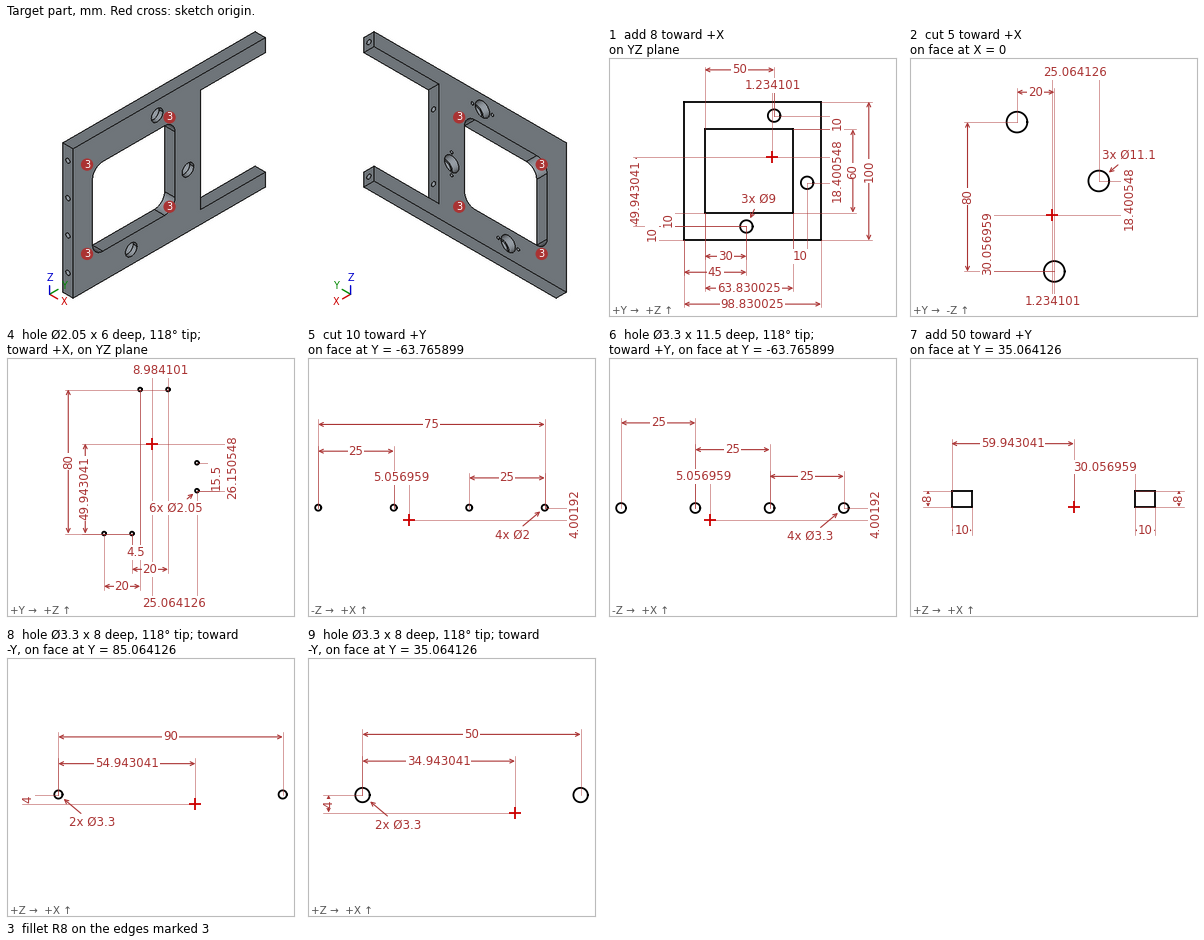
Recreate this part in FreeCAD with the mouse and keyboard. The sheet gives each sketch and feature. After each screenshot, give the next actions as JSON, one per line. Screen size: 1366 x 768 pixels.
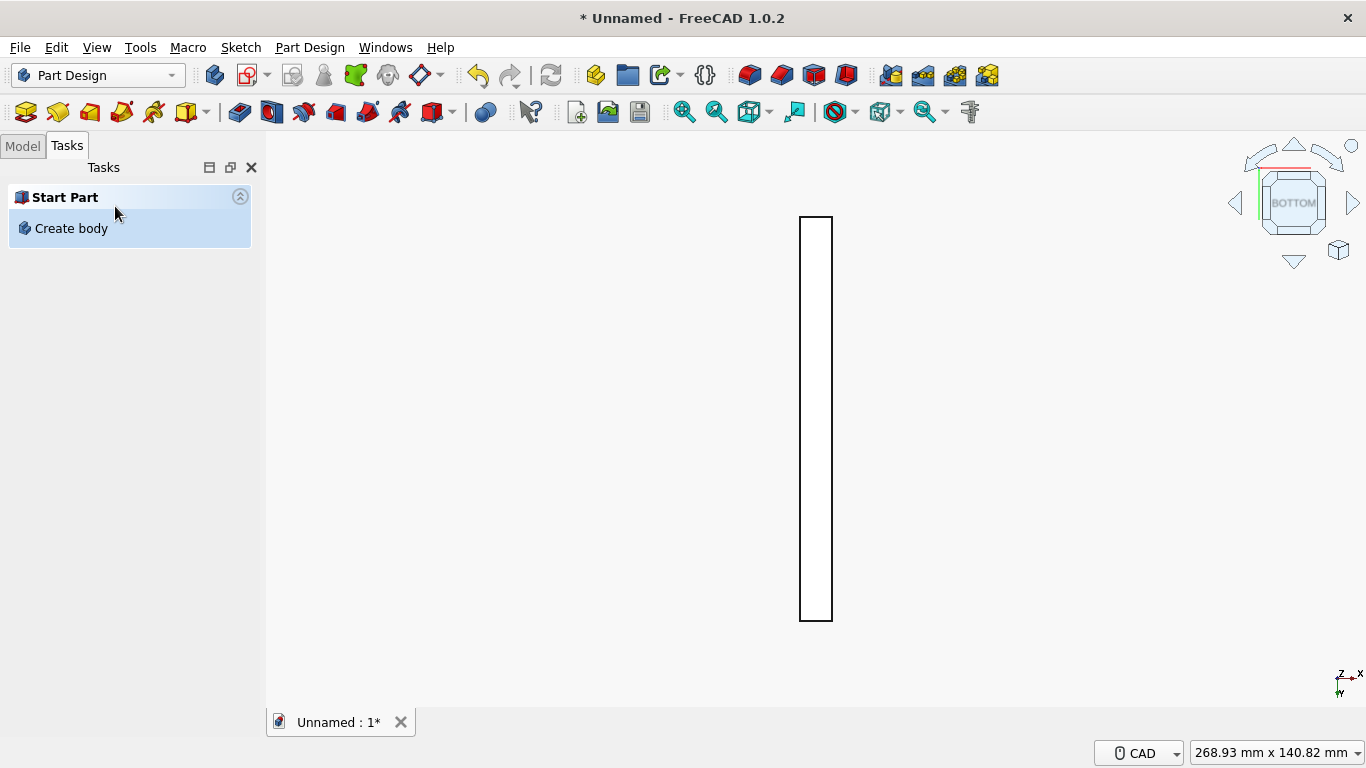
{"action": "key", "text": "4"}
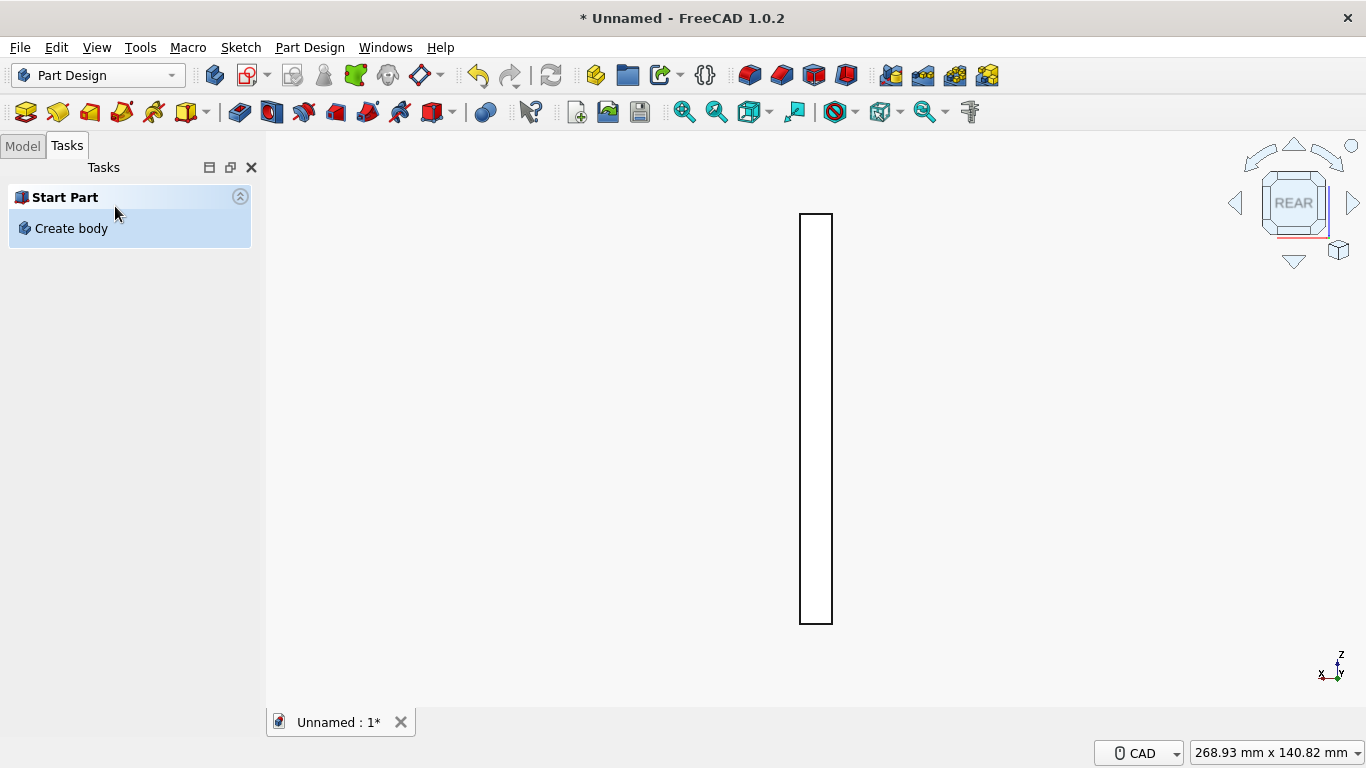
{"action": "key", "text": "6"}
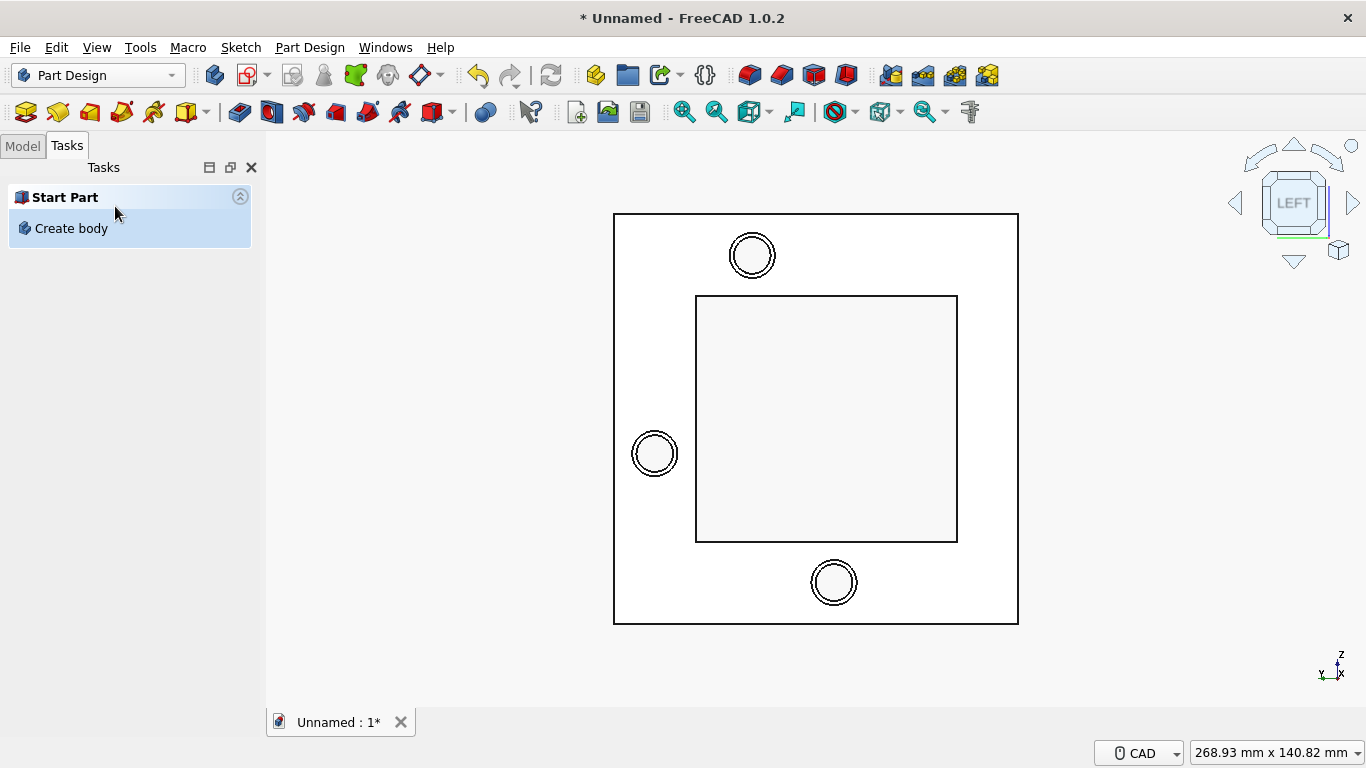
{"action": "key", "text": "v 3"}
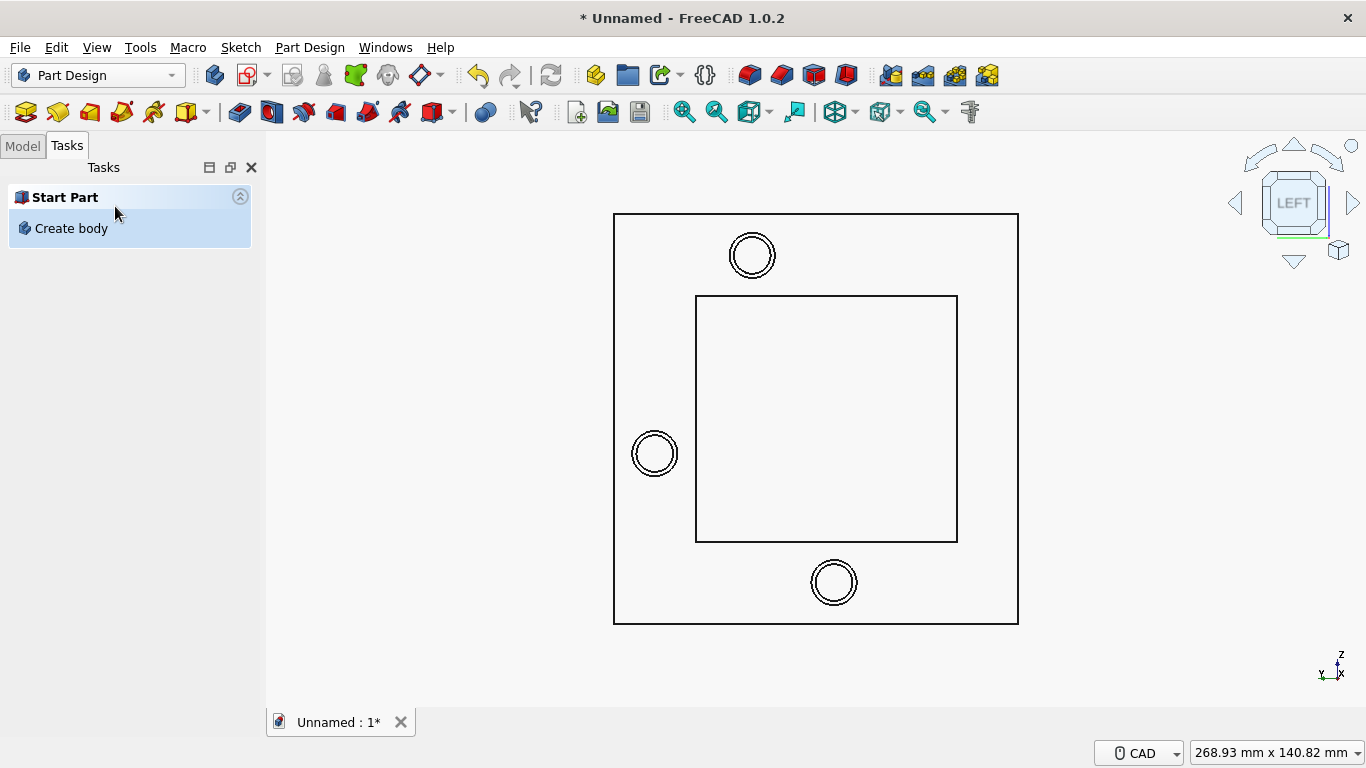
{"action": "key", "text": "0"}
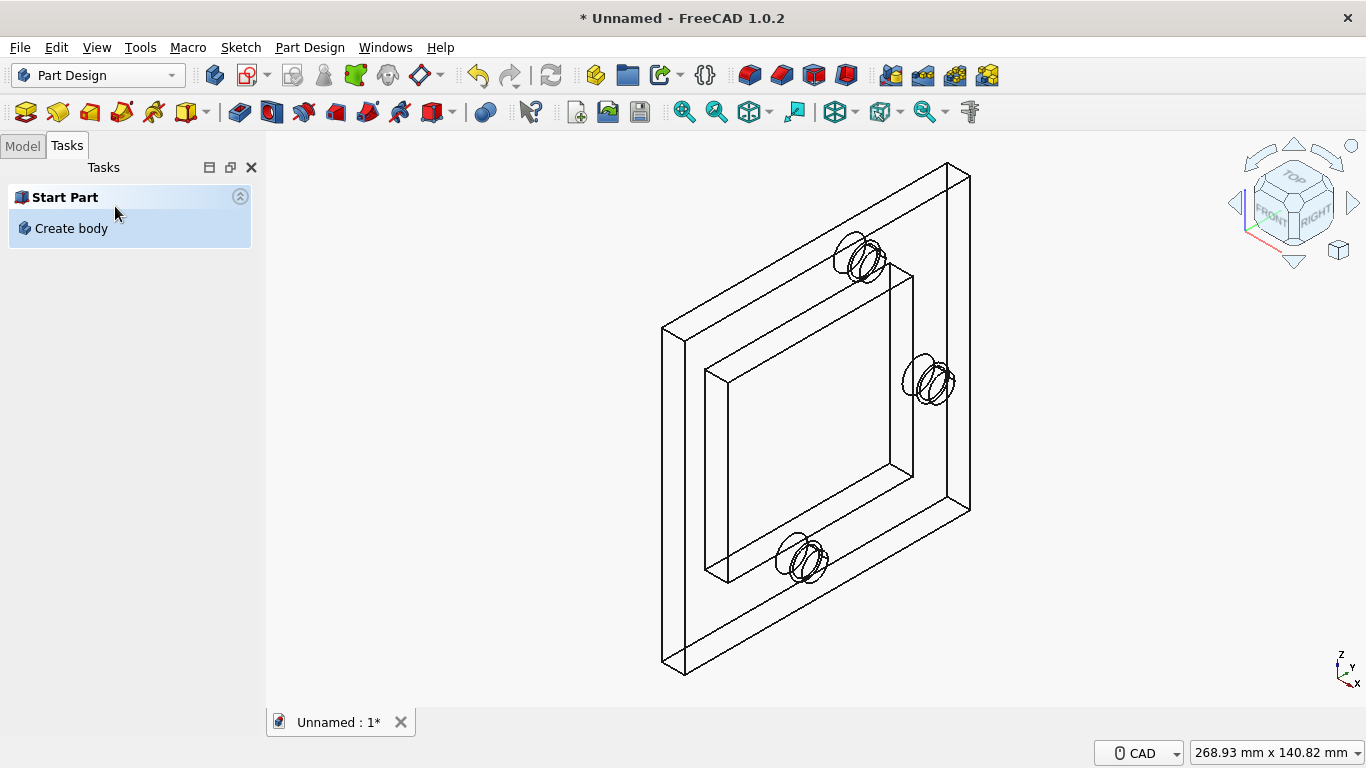
{"action": "left_click", "coordinate": [901, 269]}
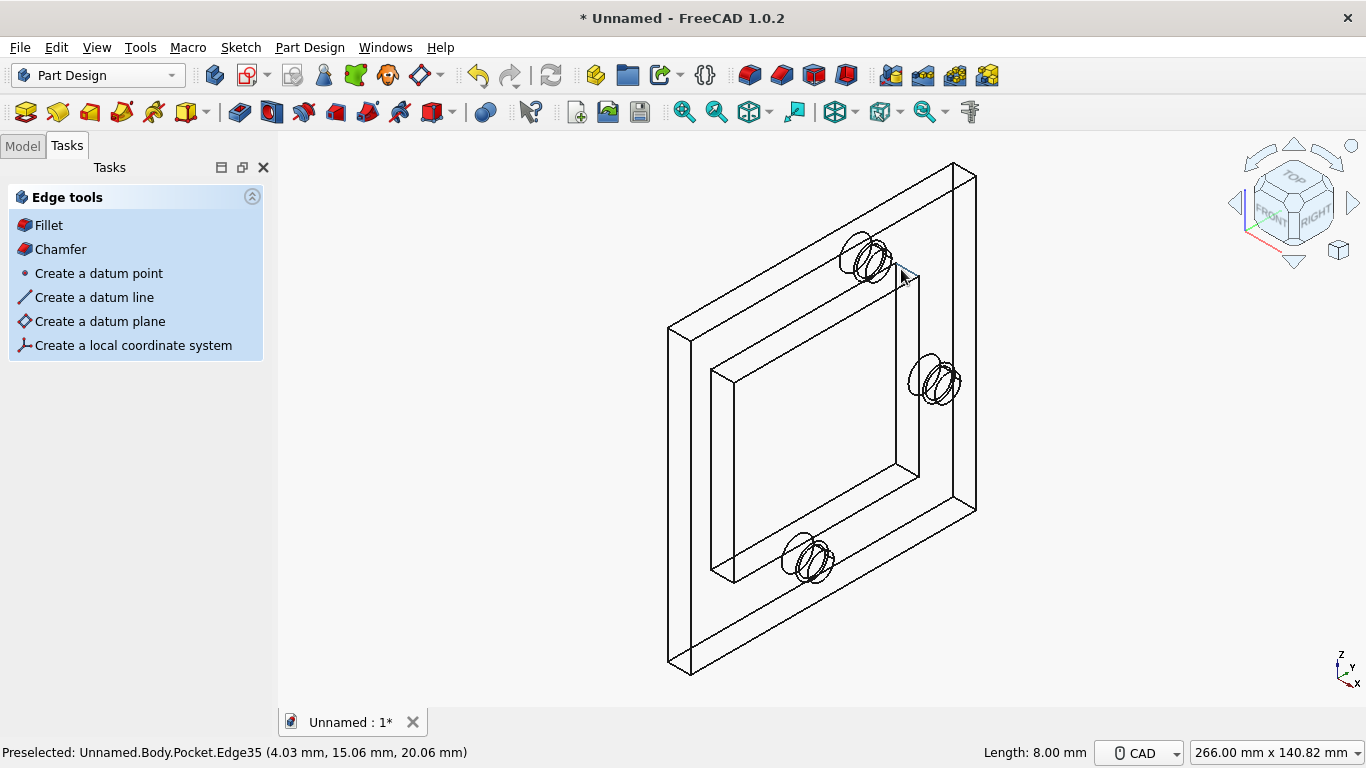
{"action": "left_click", "coordinate": [722, 375], "text": "ctrl"}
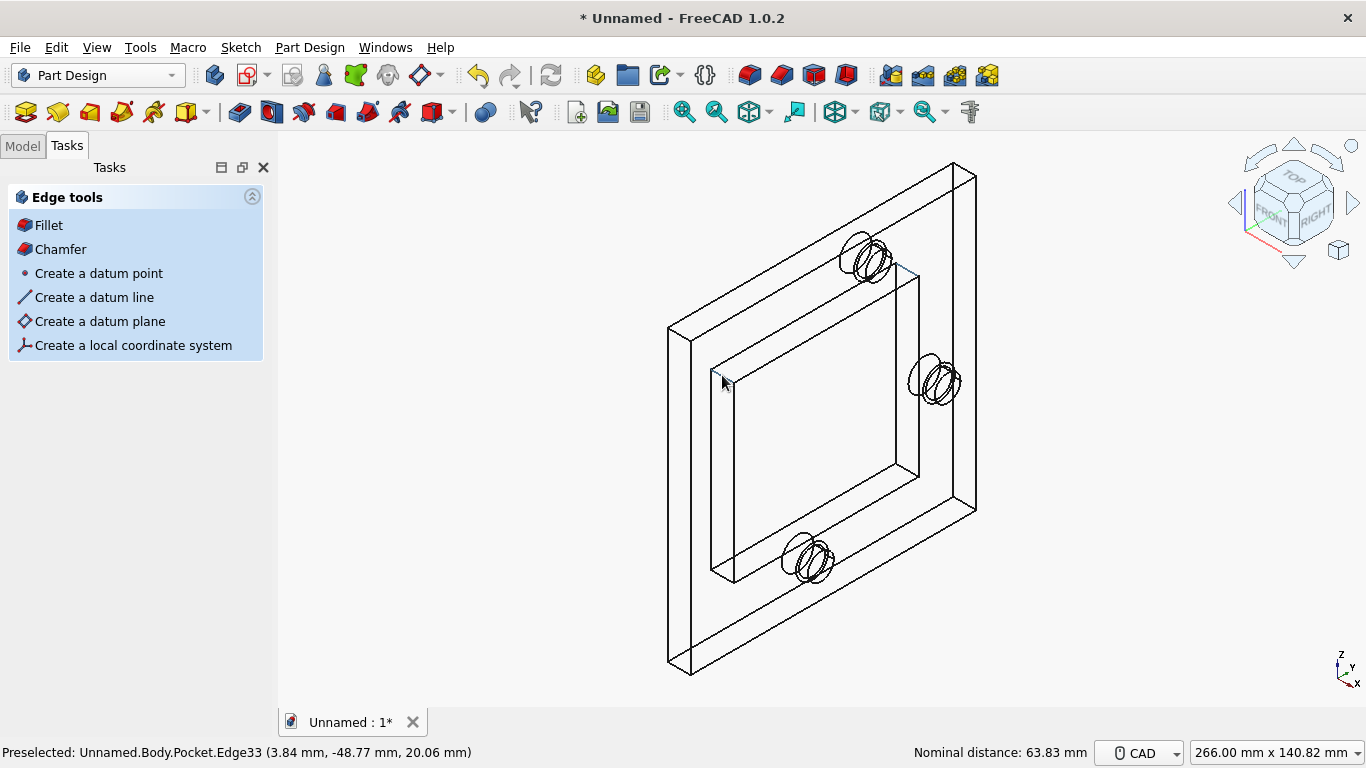
{"action": "left_click", "coordinate": [722, 576], "text": "ctrl"}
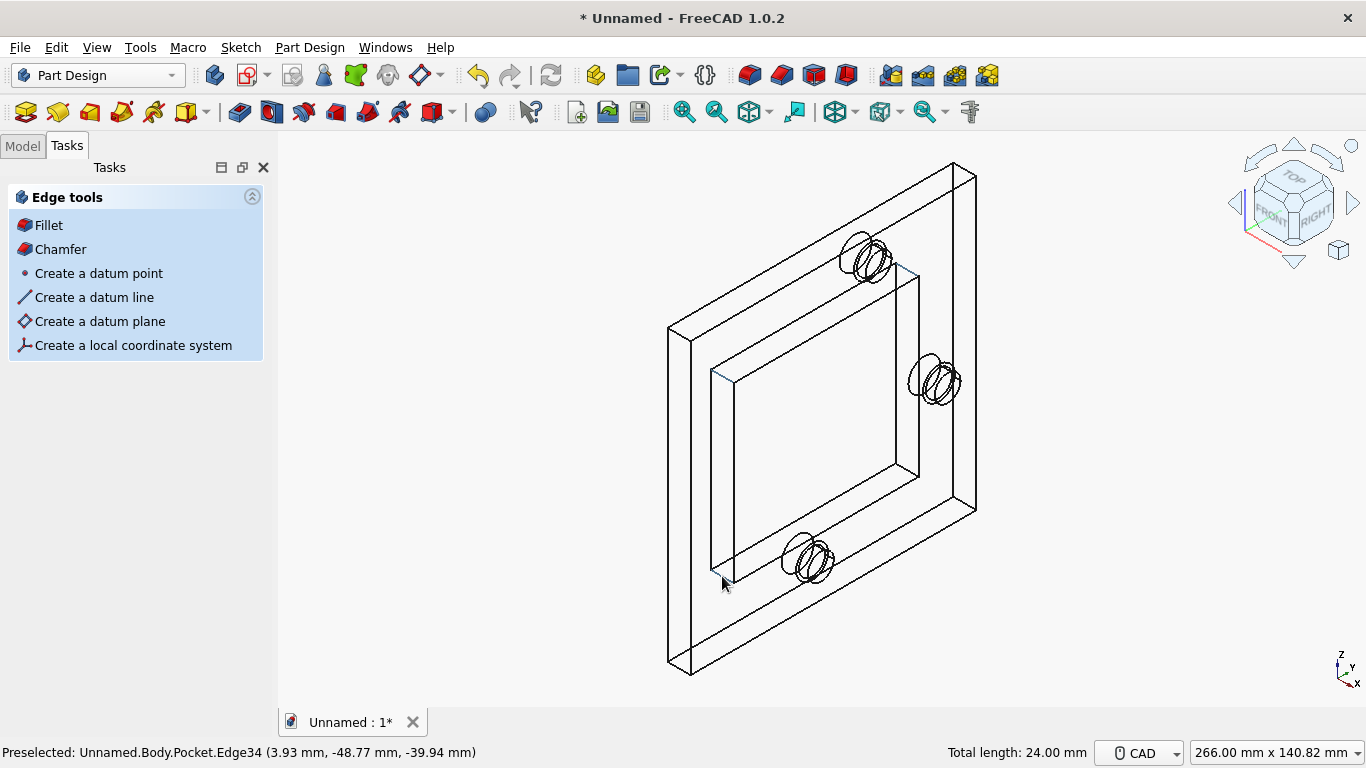
{"action": "left_click", "coordinate": [907, 469], "text": "ctrl"}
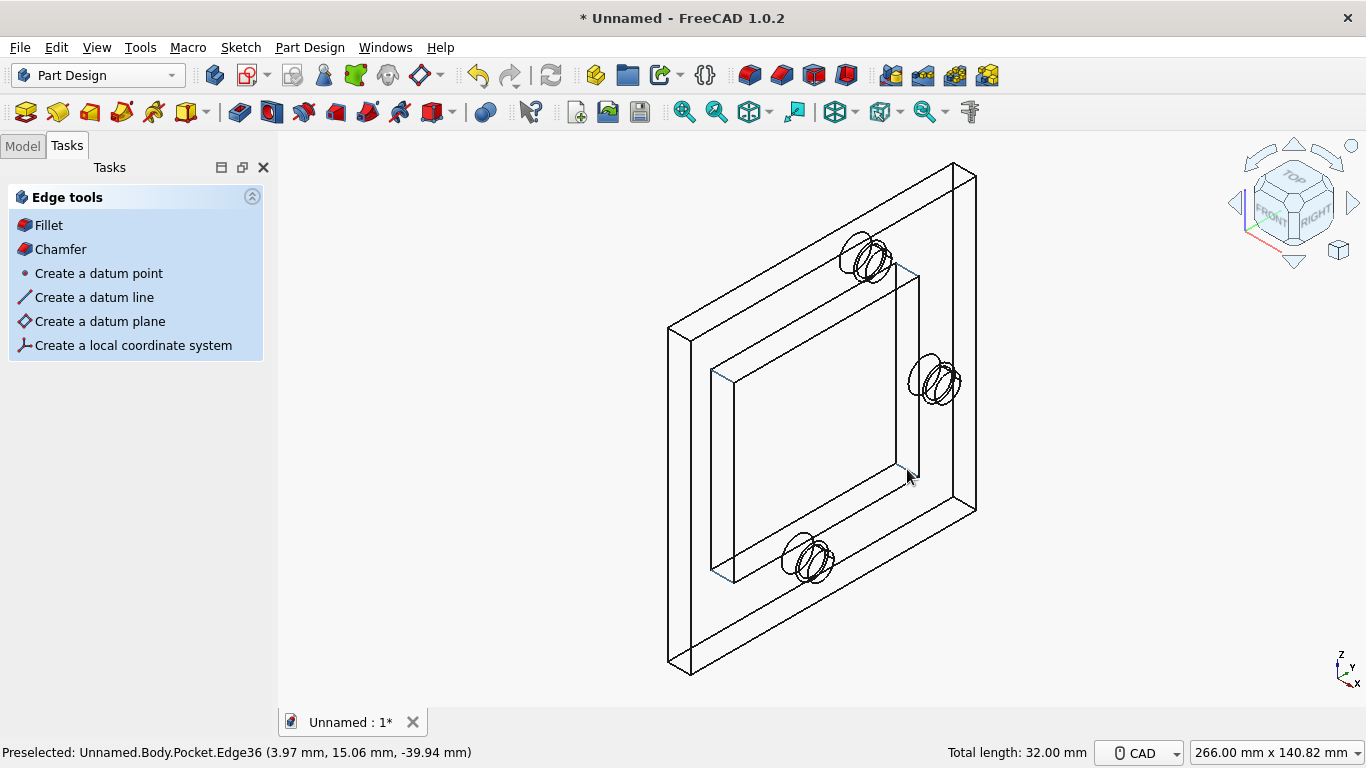
{"action": "key", "text": "v 1"}